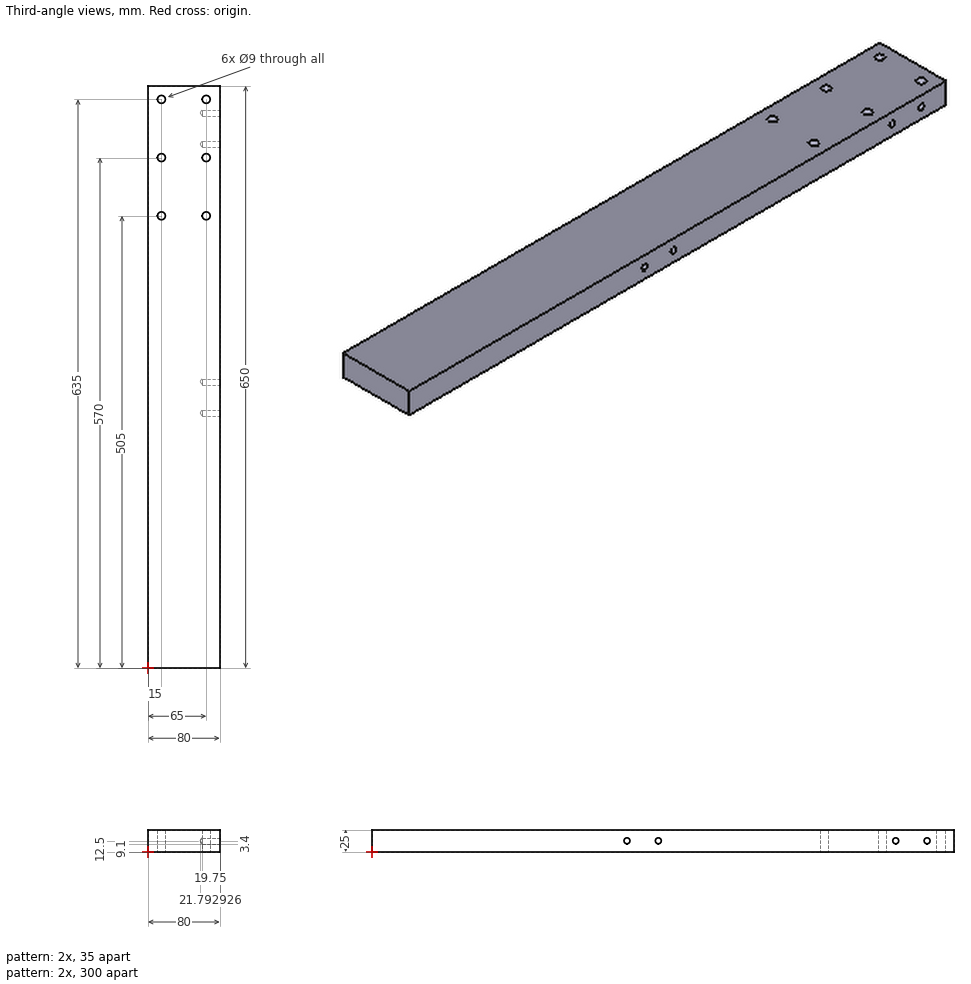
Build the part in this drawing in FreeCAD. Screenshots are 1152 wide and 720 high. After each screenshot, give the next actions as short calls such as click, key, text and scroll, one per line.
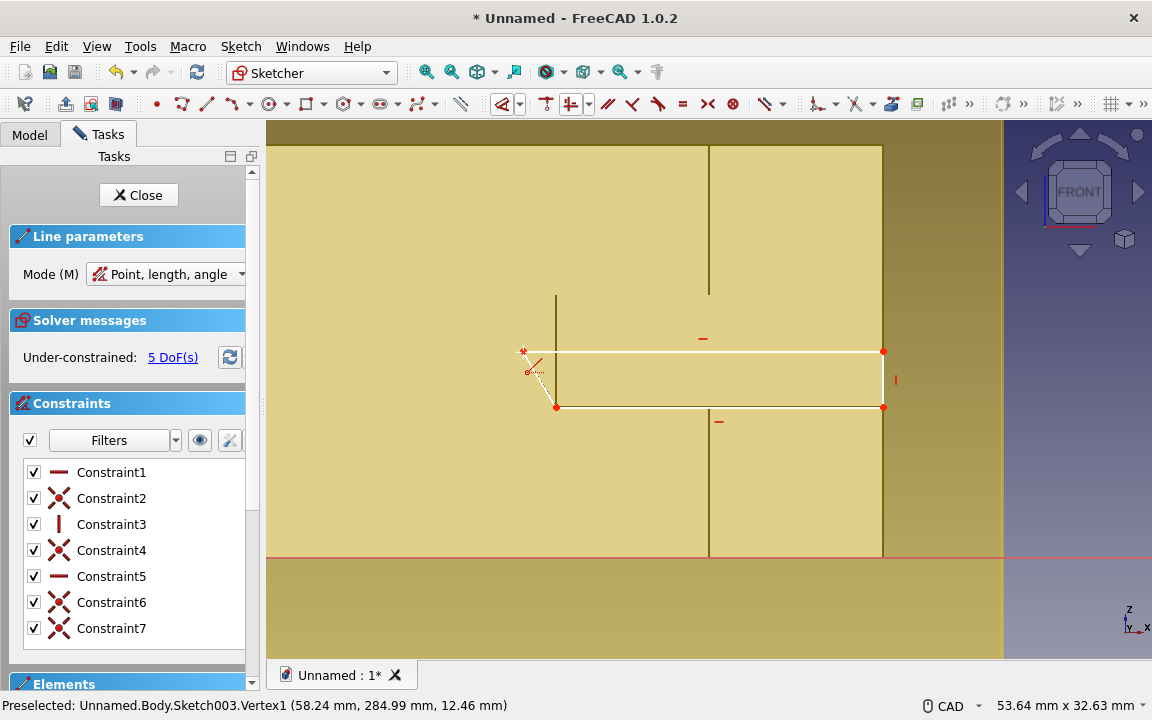
click(487, 351)
click(379, 351)
key(Escape)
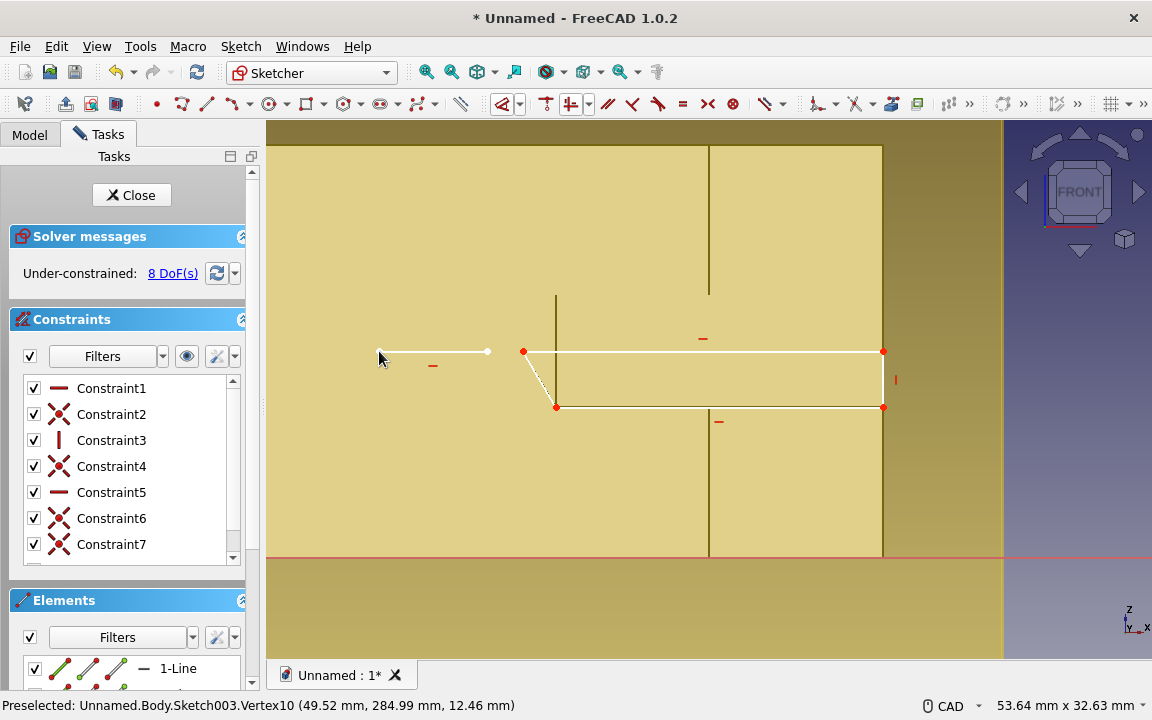
click(455, 352)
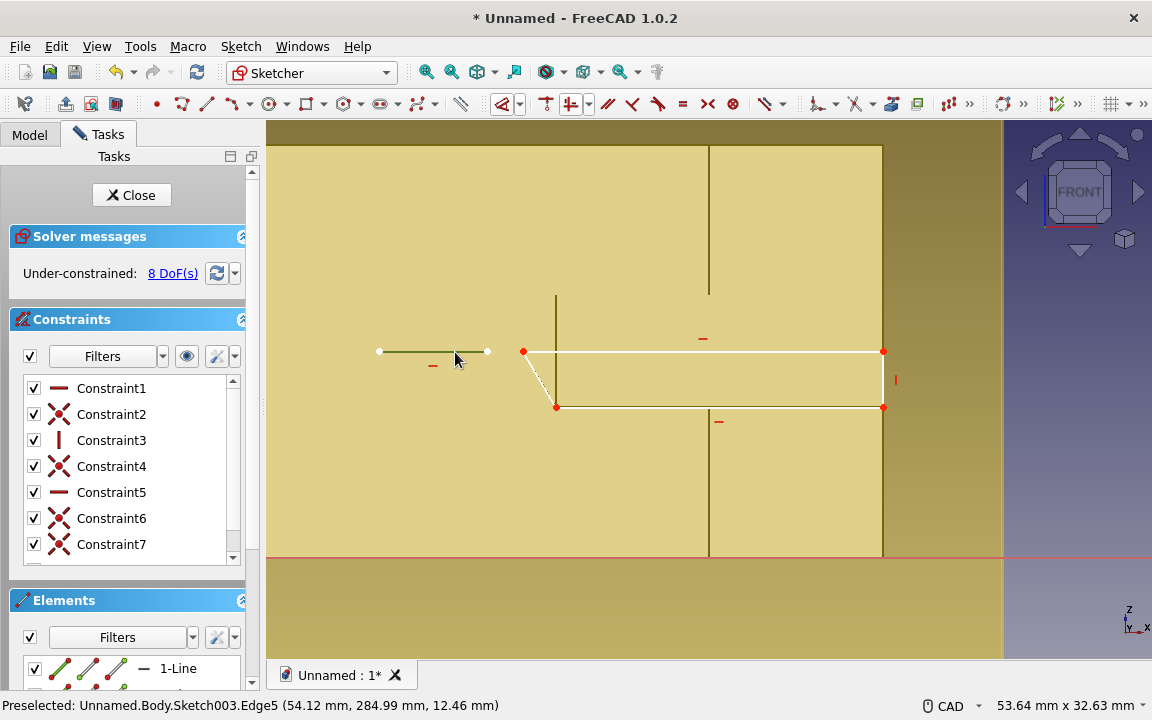
click(461, 104)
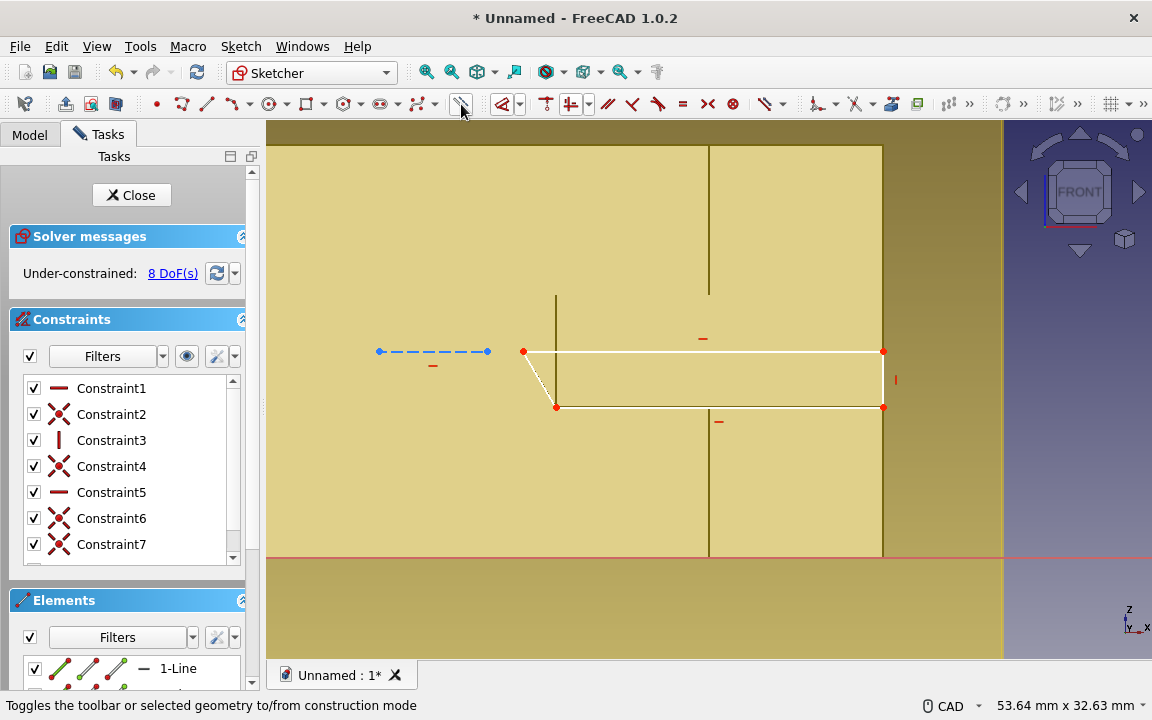
click(502, 104)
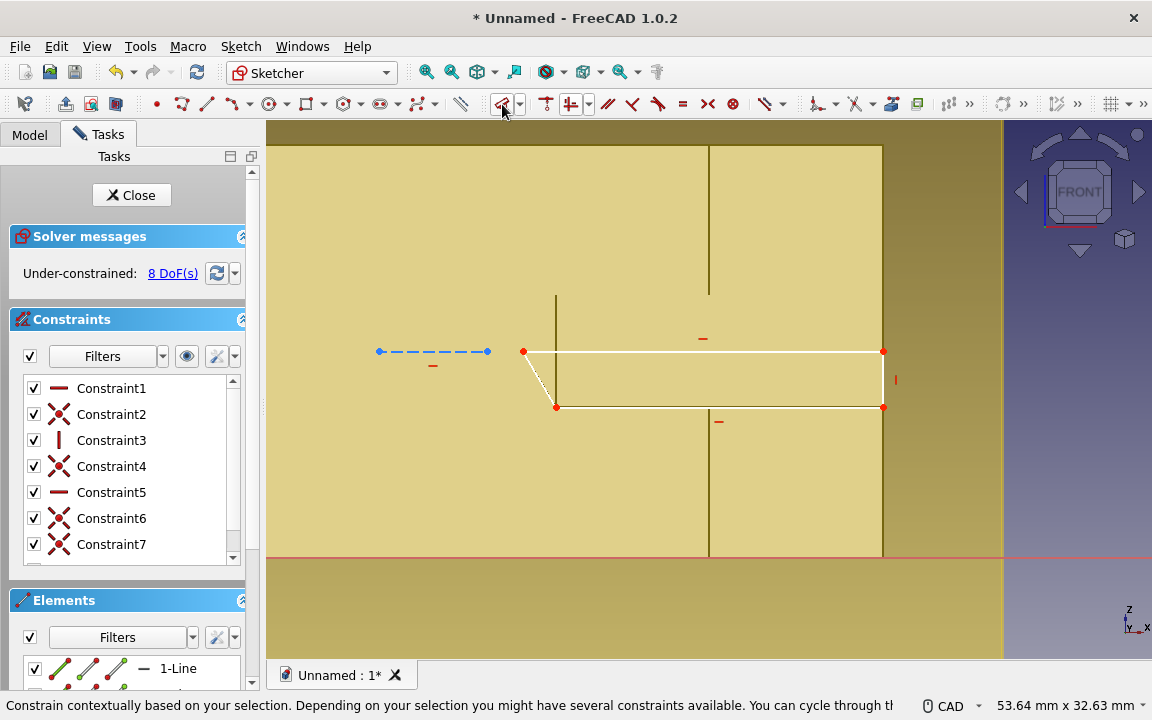
click(883, 369)
click(917, 380)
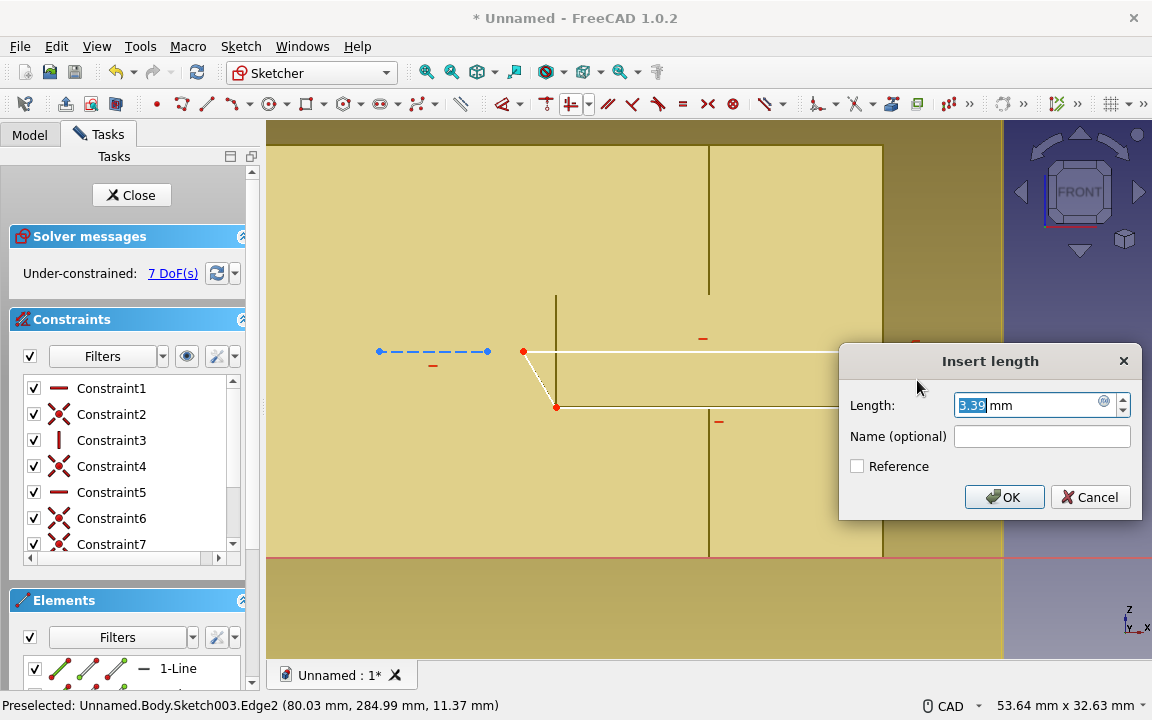
text(3.4)
key(Return)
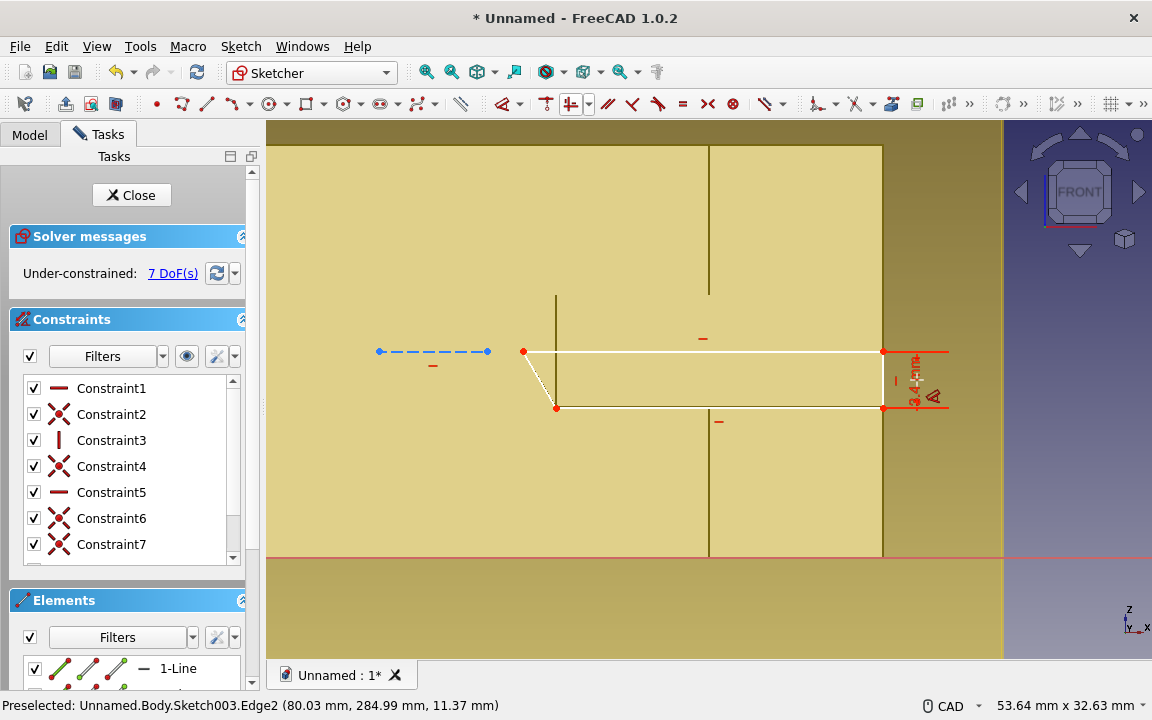
click(883, 352)
click(588, 592)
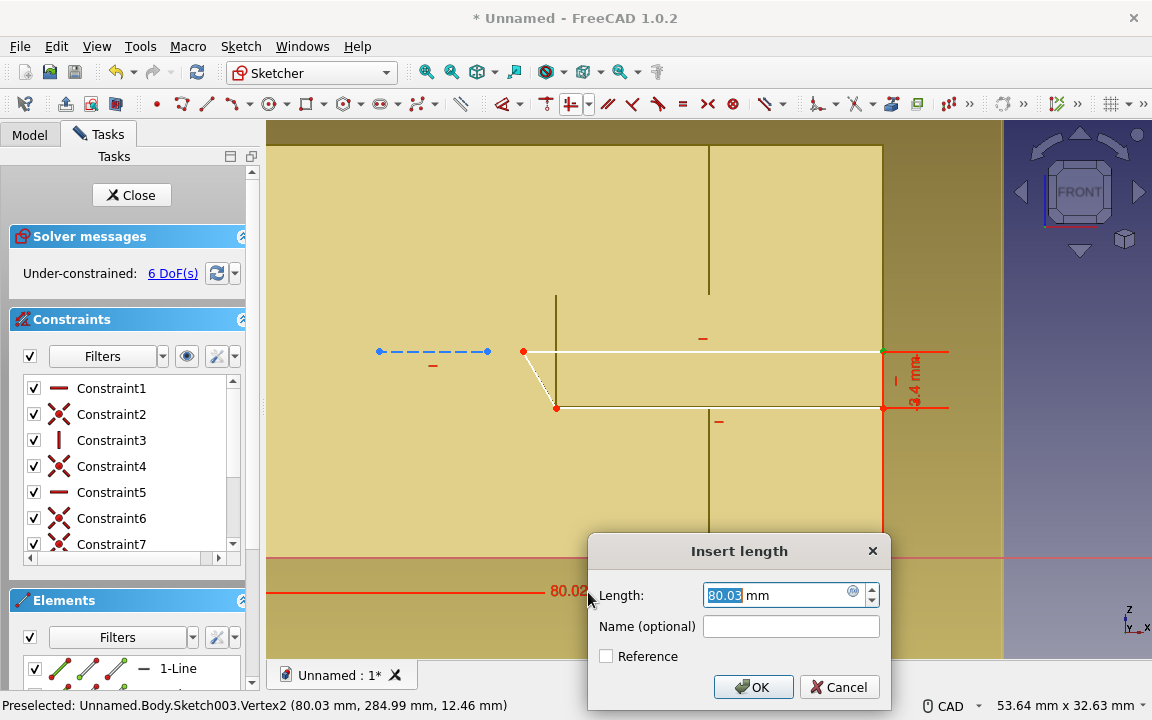
text(80)
key(Return)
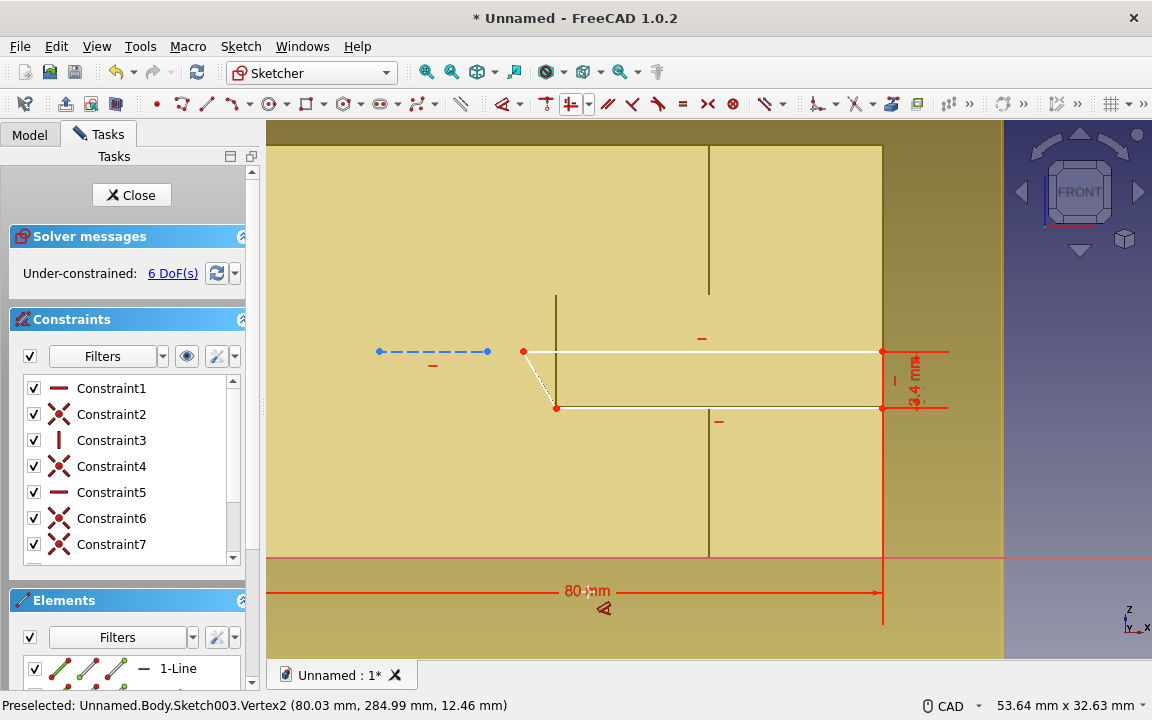
click(883, 408)
click(917, 483)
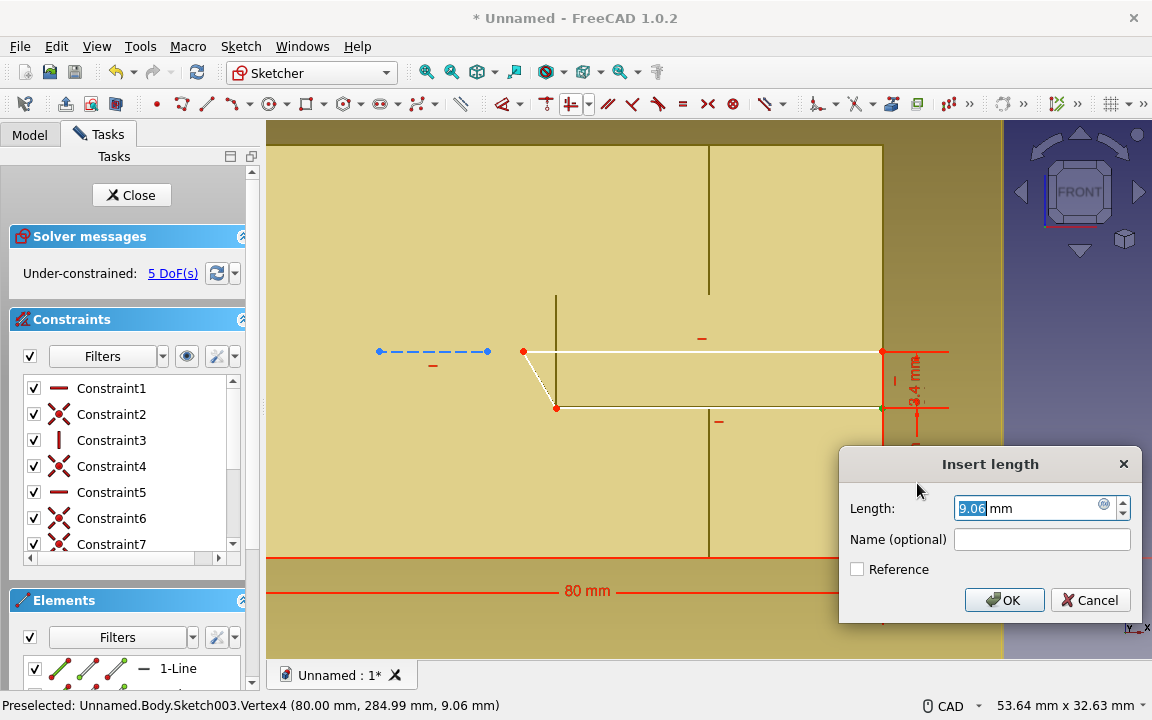
text(9.1)
key(Return)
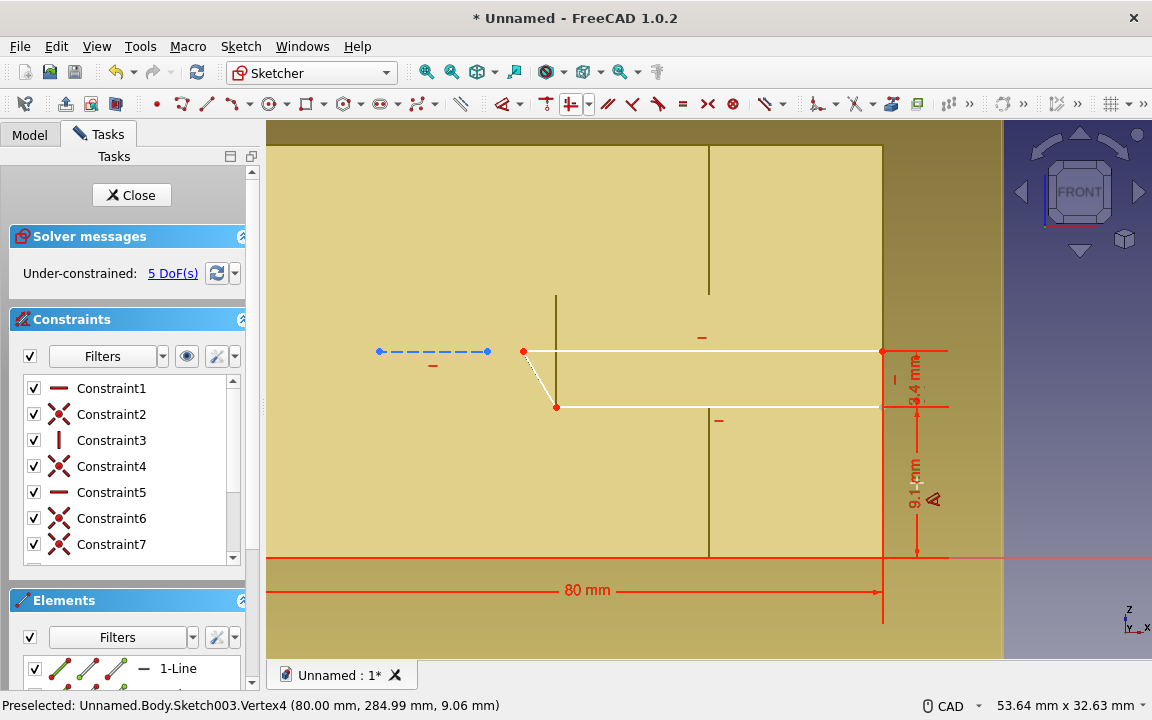
click(785, 407)
click(719, 441)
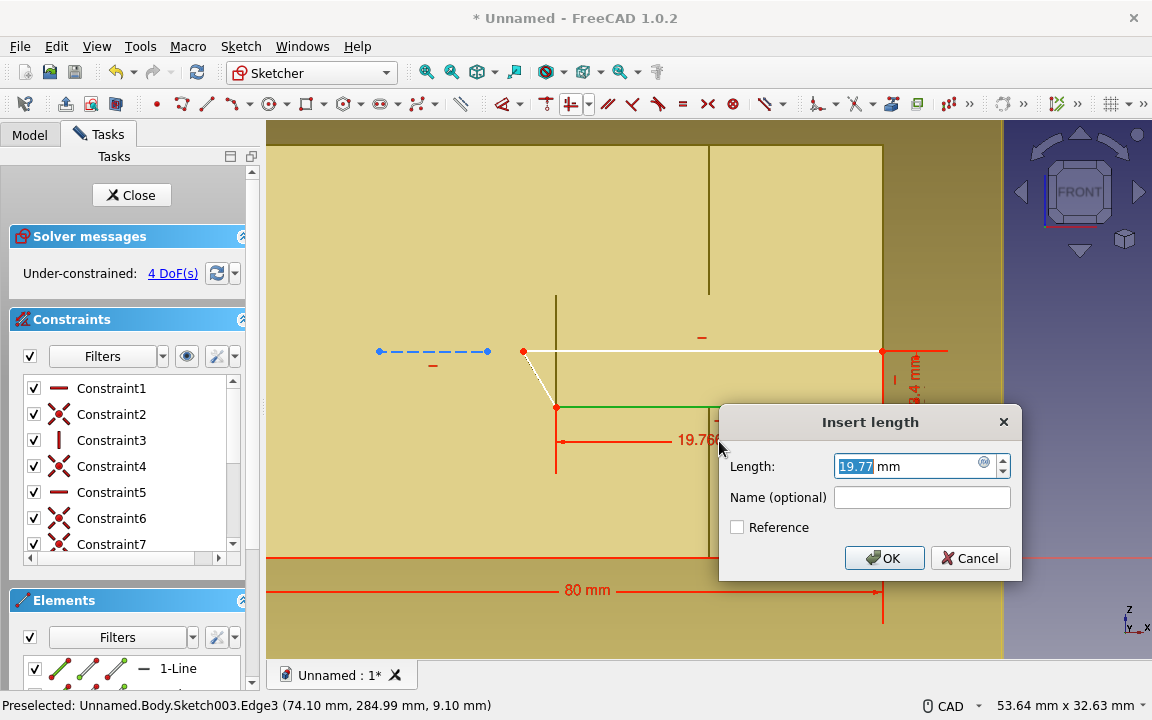
text(19.75)
key(Return)